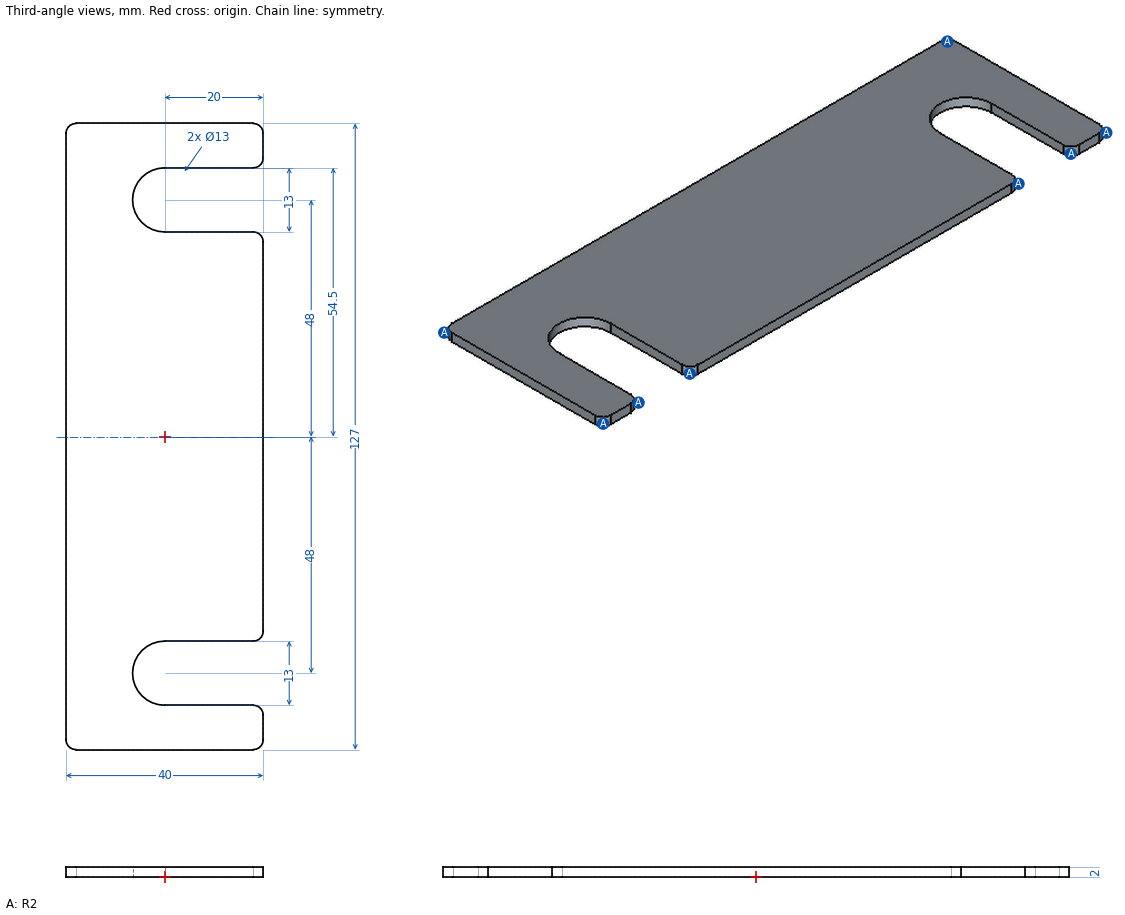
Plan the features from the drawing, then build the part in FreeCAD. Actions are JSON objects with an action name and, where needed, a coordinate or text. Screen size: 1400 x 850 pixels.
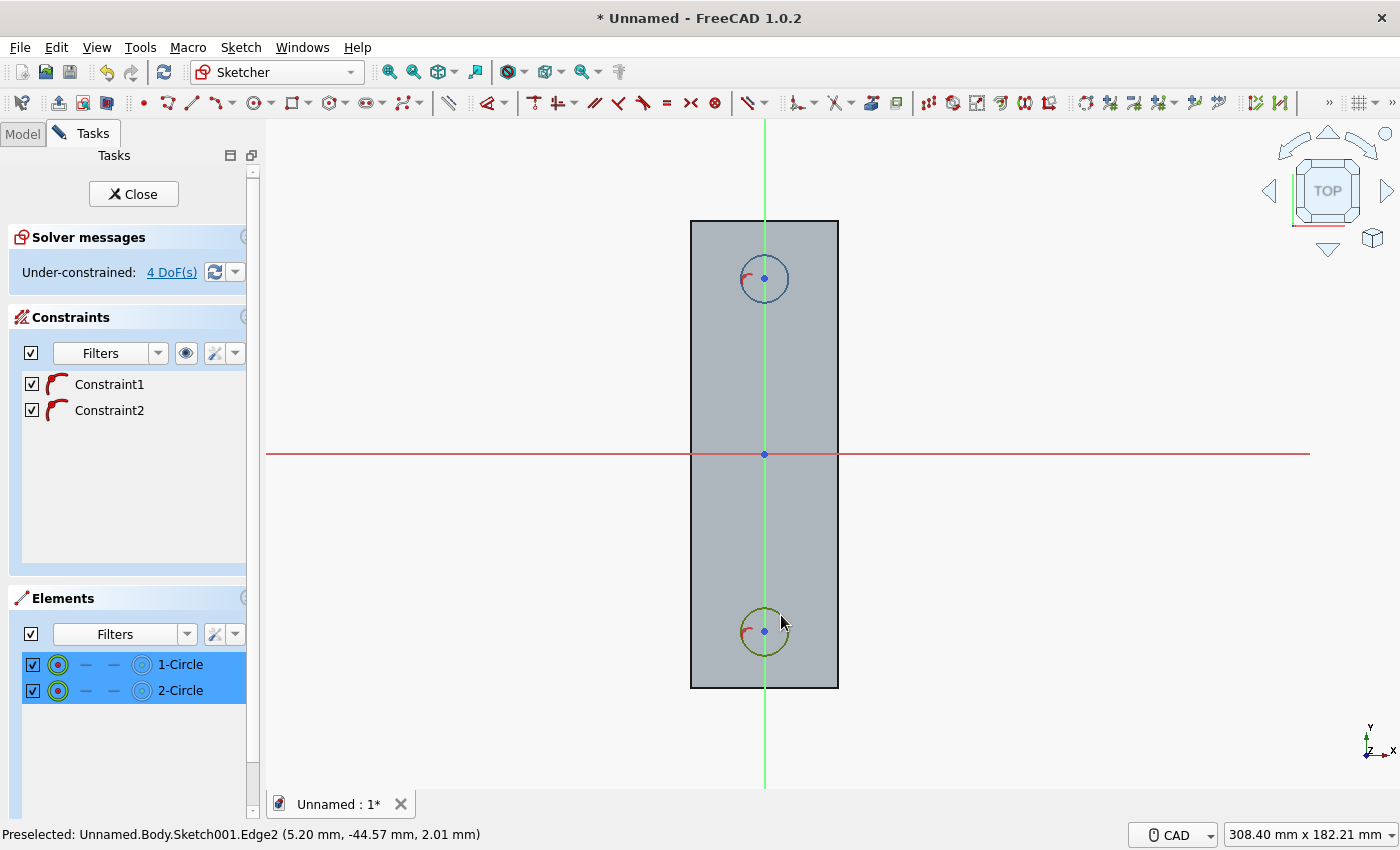
{"action": "left_click", "coordinate": [668, 104]}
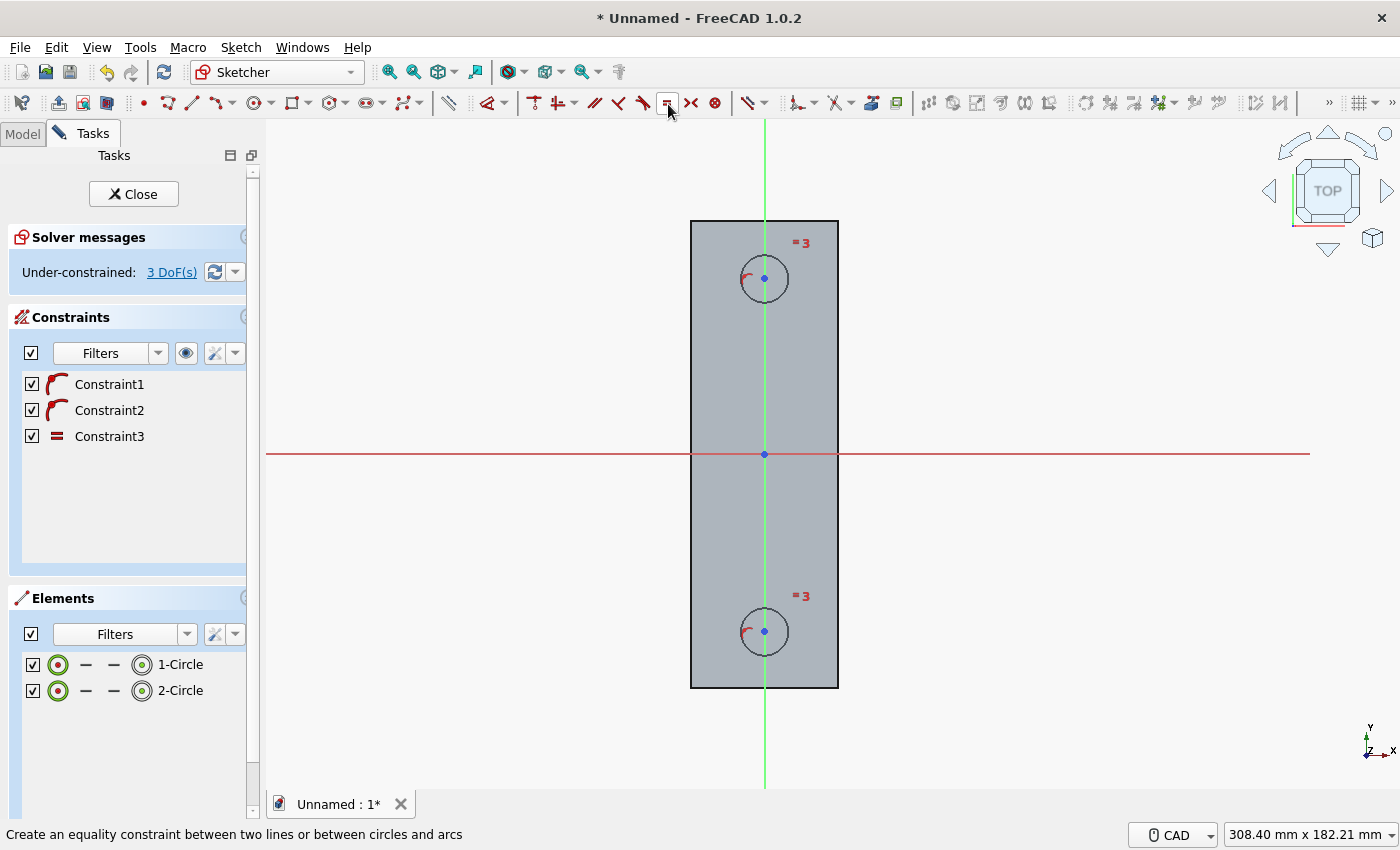
{"action": "left_click", "coordinate": [488, 104]}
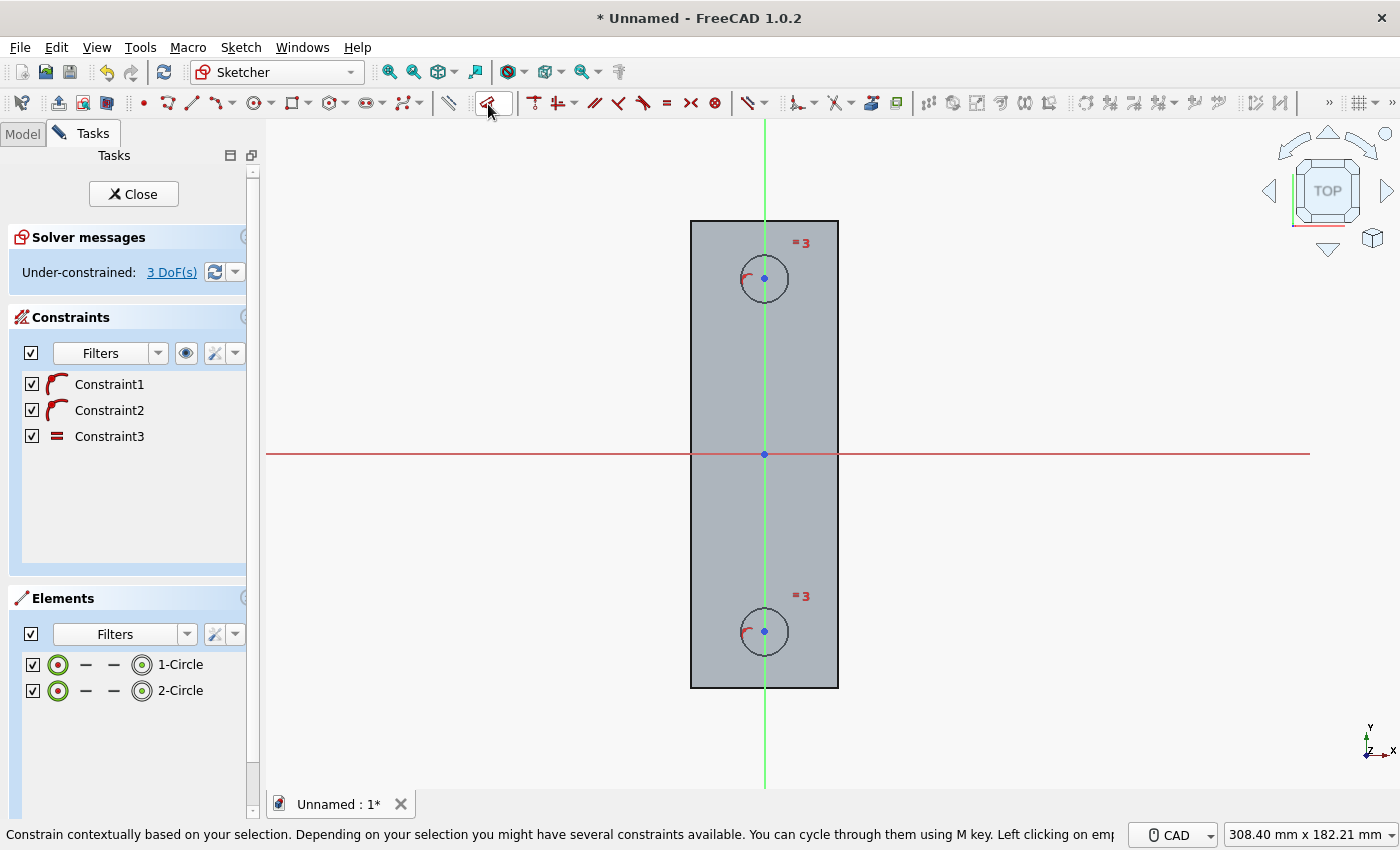
{"action": "left_click", "coordinate": [781, 262]}
{"action": "left_click", "coordinate": [803, 239]}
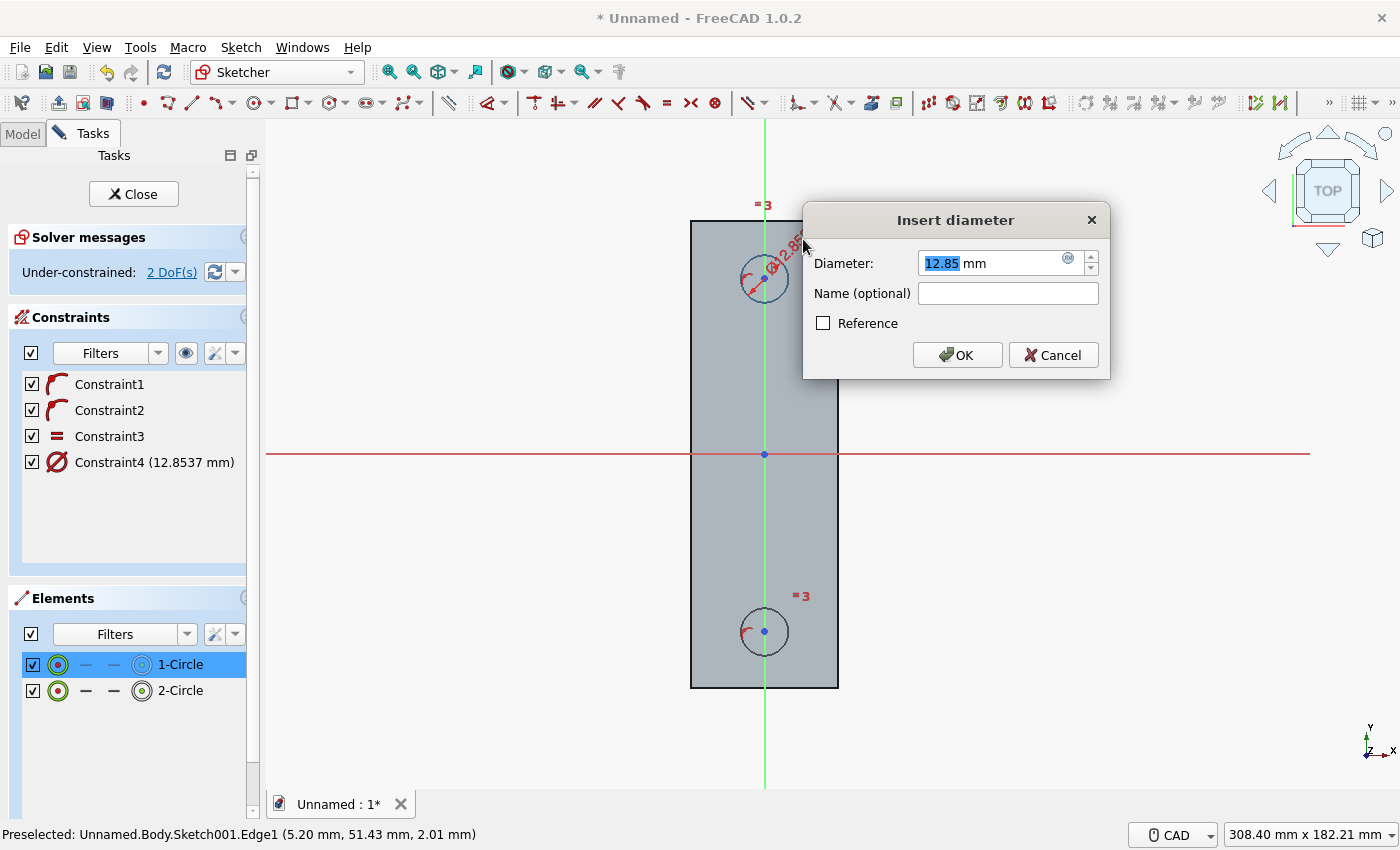
{"action": "type", "text": "13"}
{"action": "key", "text": "Return"}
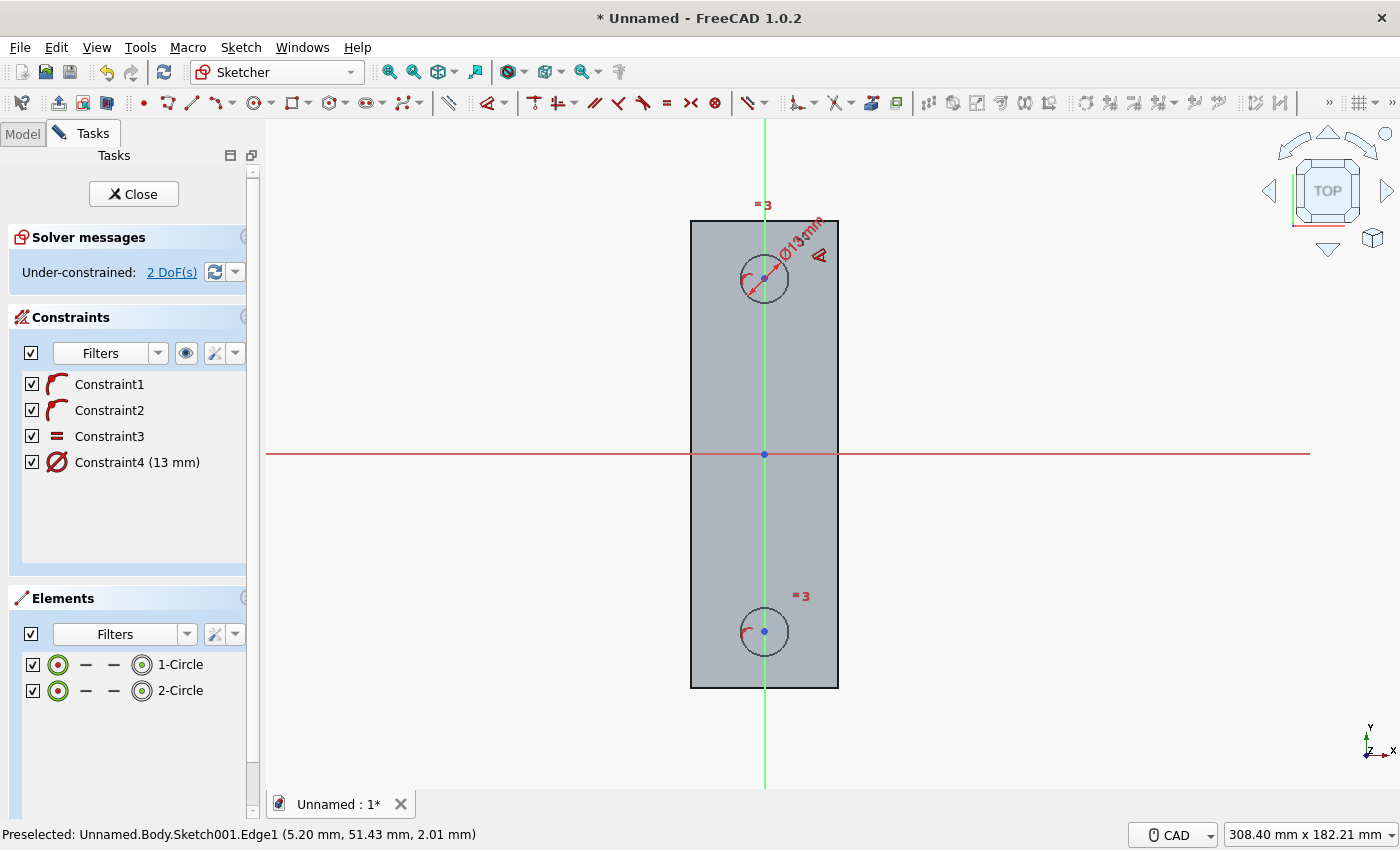
{"action": "left_click", "coordinate": [765, 279]}
{"action": "left_click", "coordinate": [799, 367]}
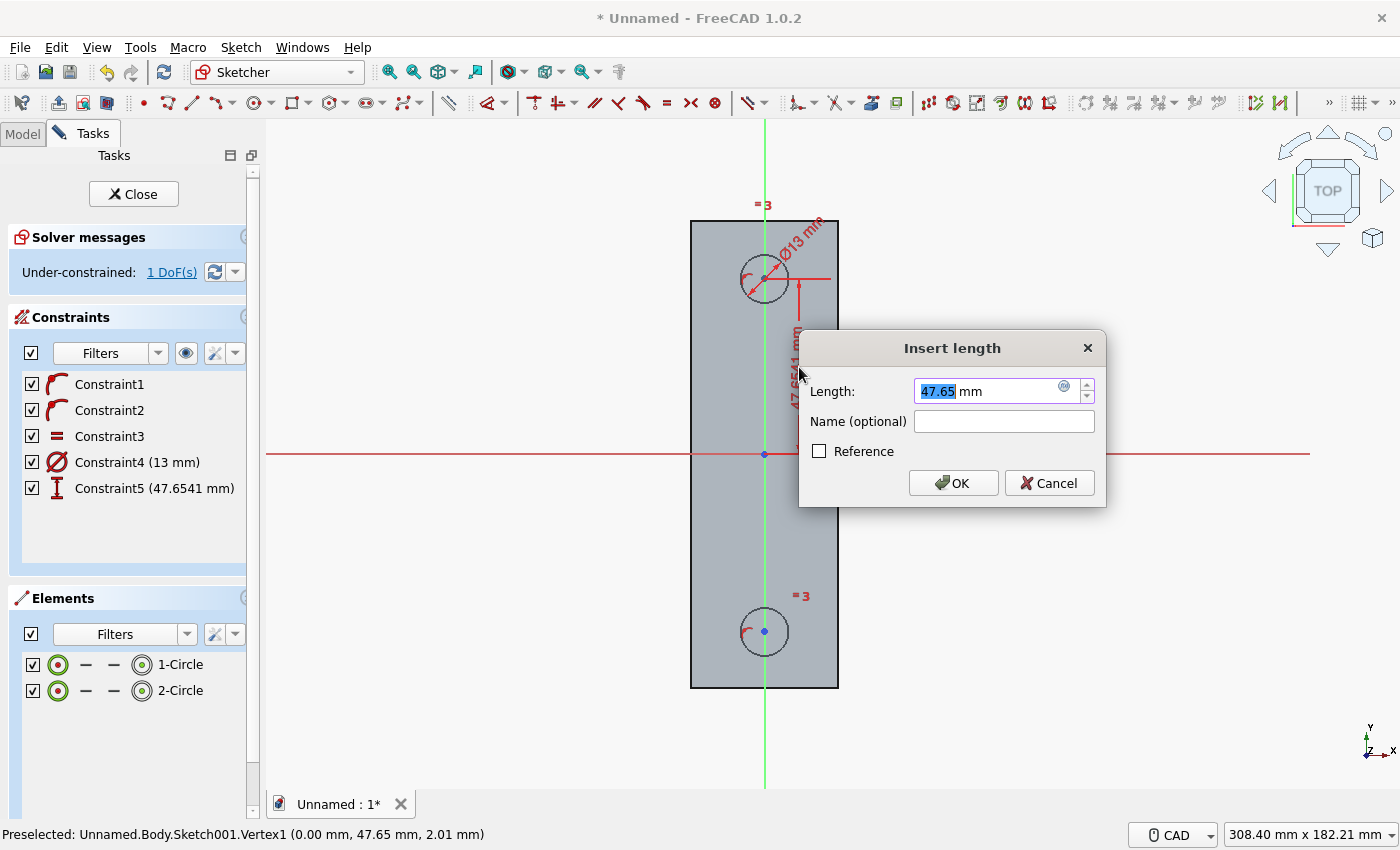
{"action": "type", "text": "48"}
{"action": "key", "text": "Return"}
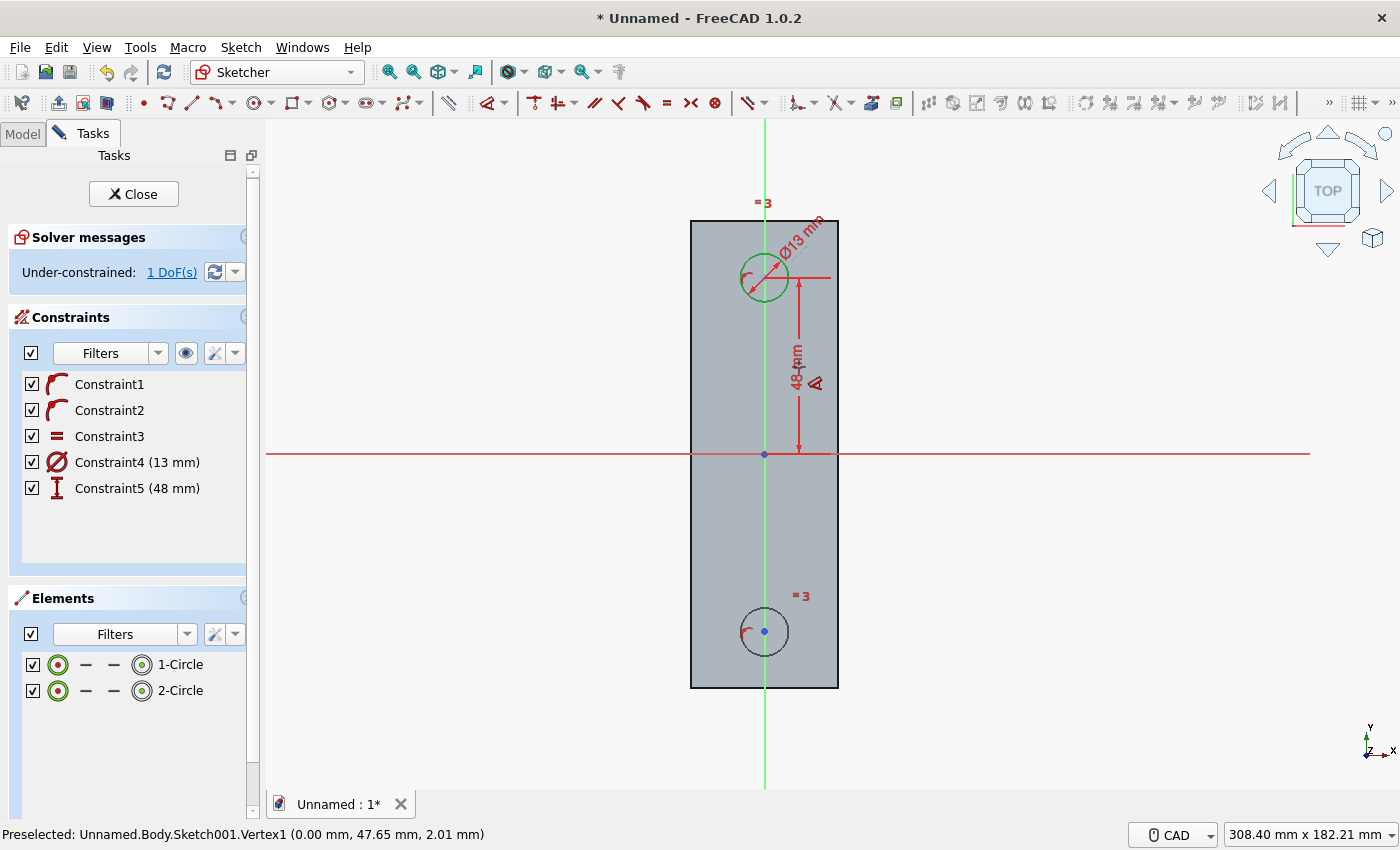
{"action": "left_click", "coordinate": [765, 632]}
{"action": "left_click", "coordinate": [799, 543]}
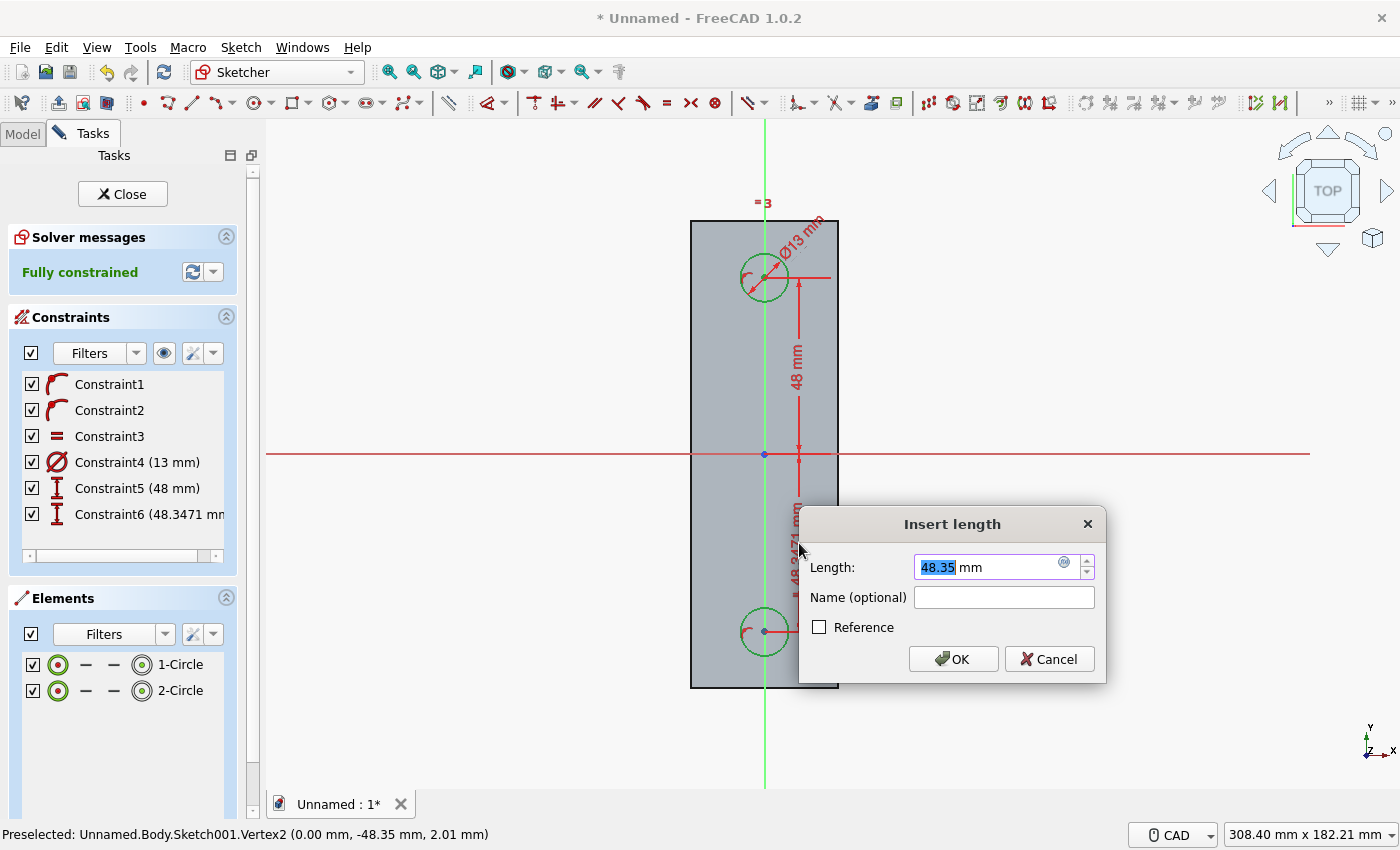
{"action": "type", "text": "48"}
{"action": "key", "text": "Return"}
{"action": "key", "text": "Escape"}